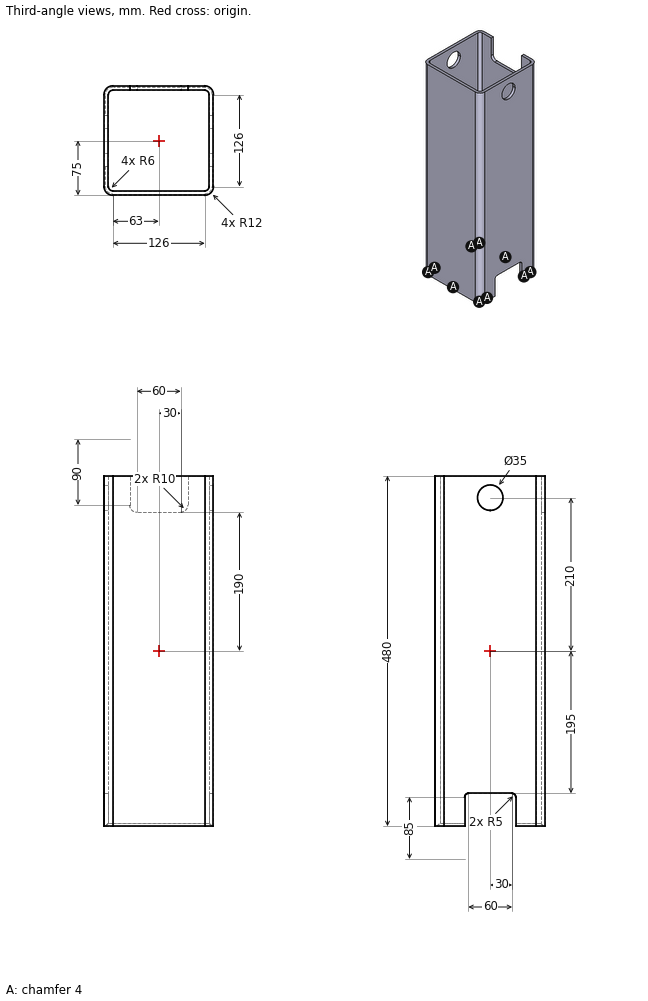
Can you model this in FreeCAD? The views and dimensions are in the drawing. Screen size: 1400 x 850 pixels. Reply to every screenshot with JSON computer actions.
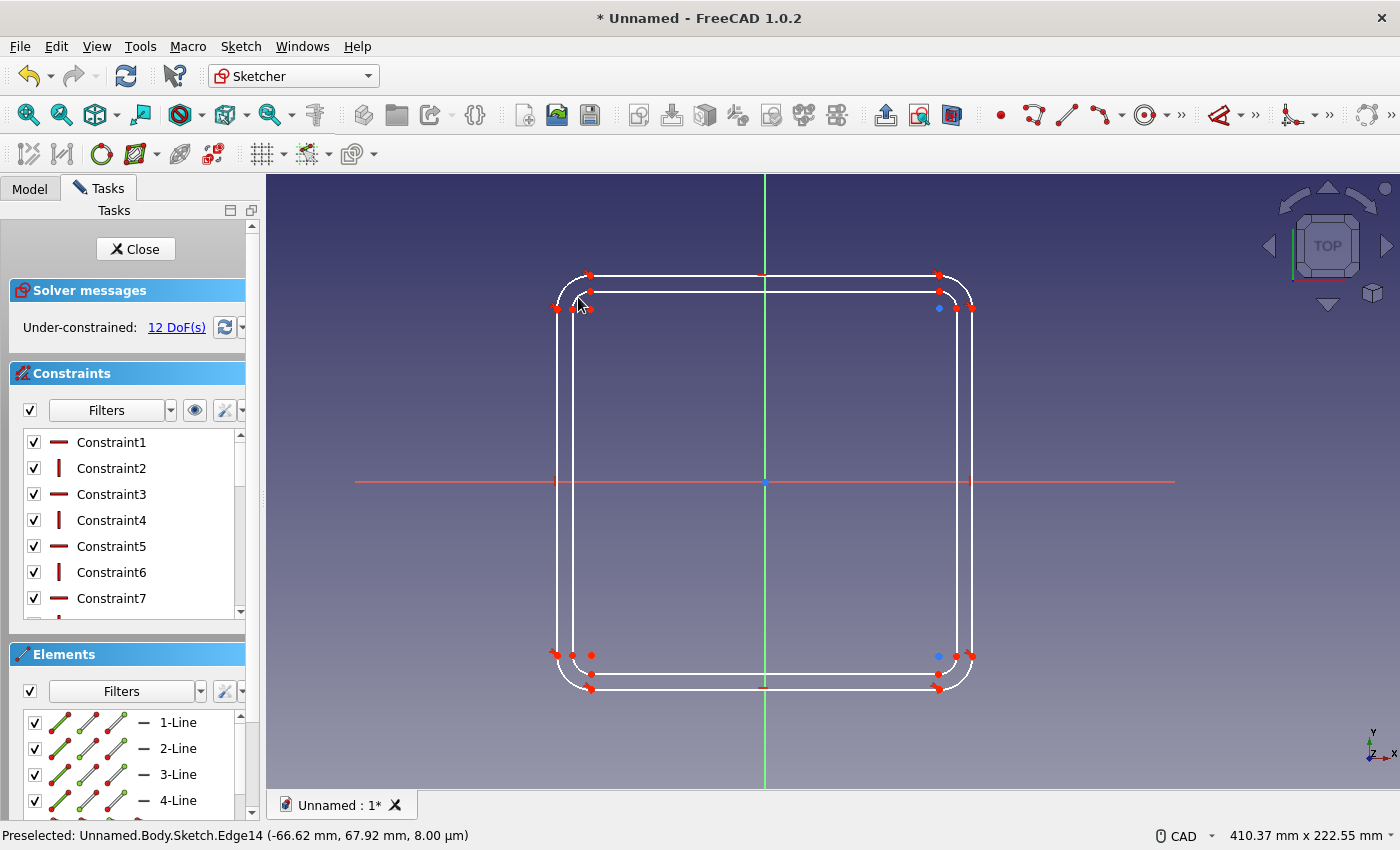
{"action": "left_click", "coordinate": [969, 294]}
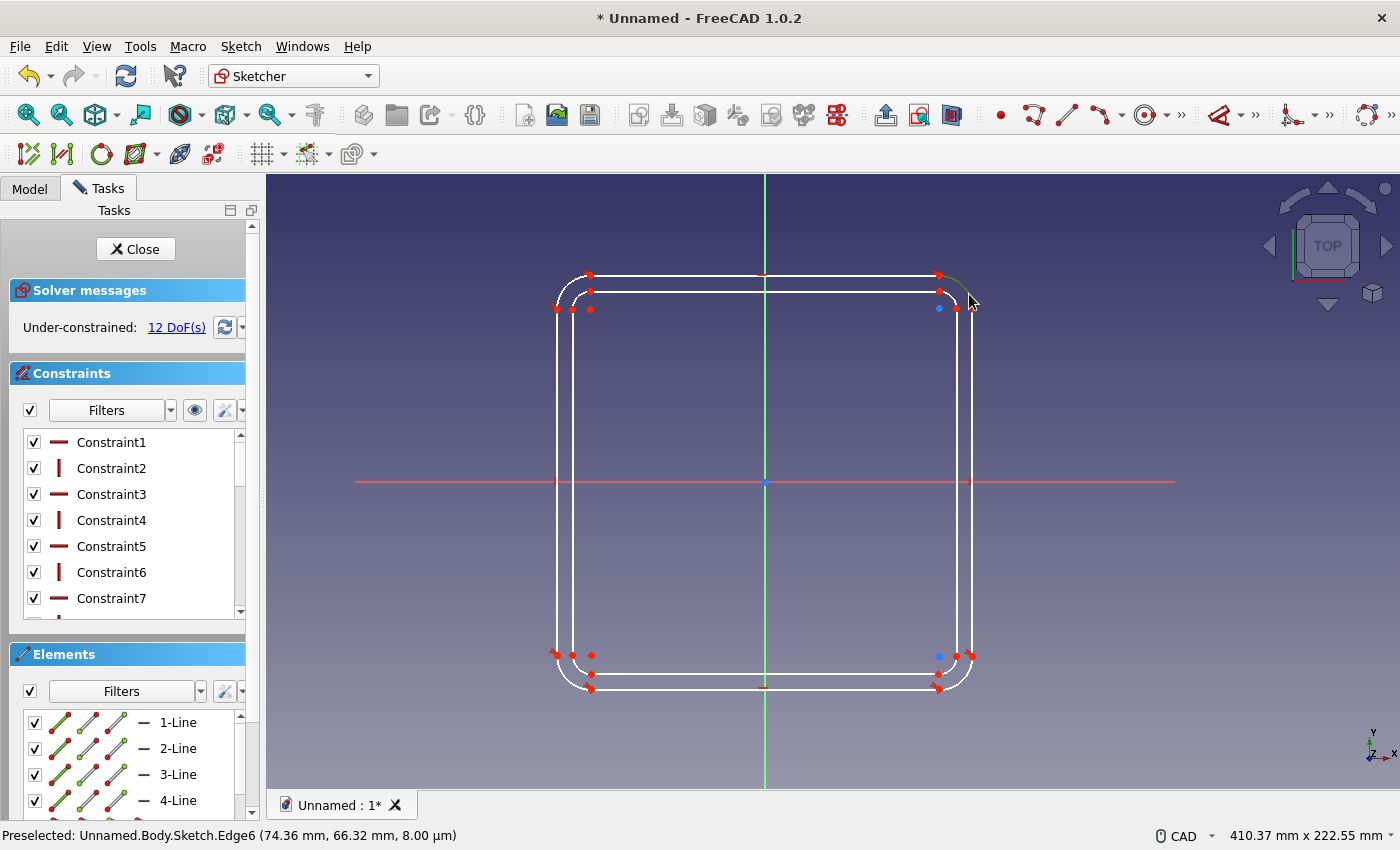
{"action": "left_click", "coordinate": [952, 297]}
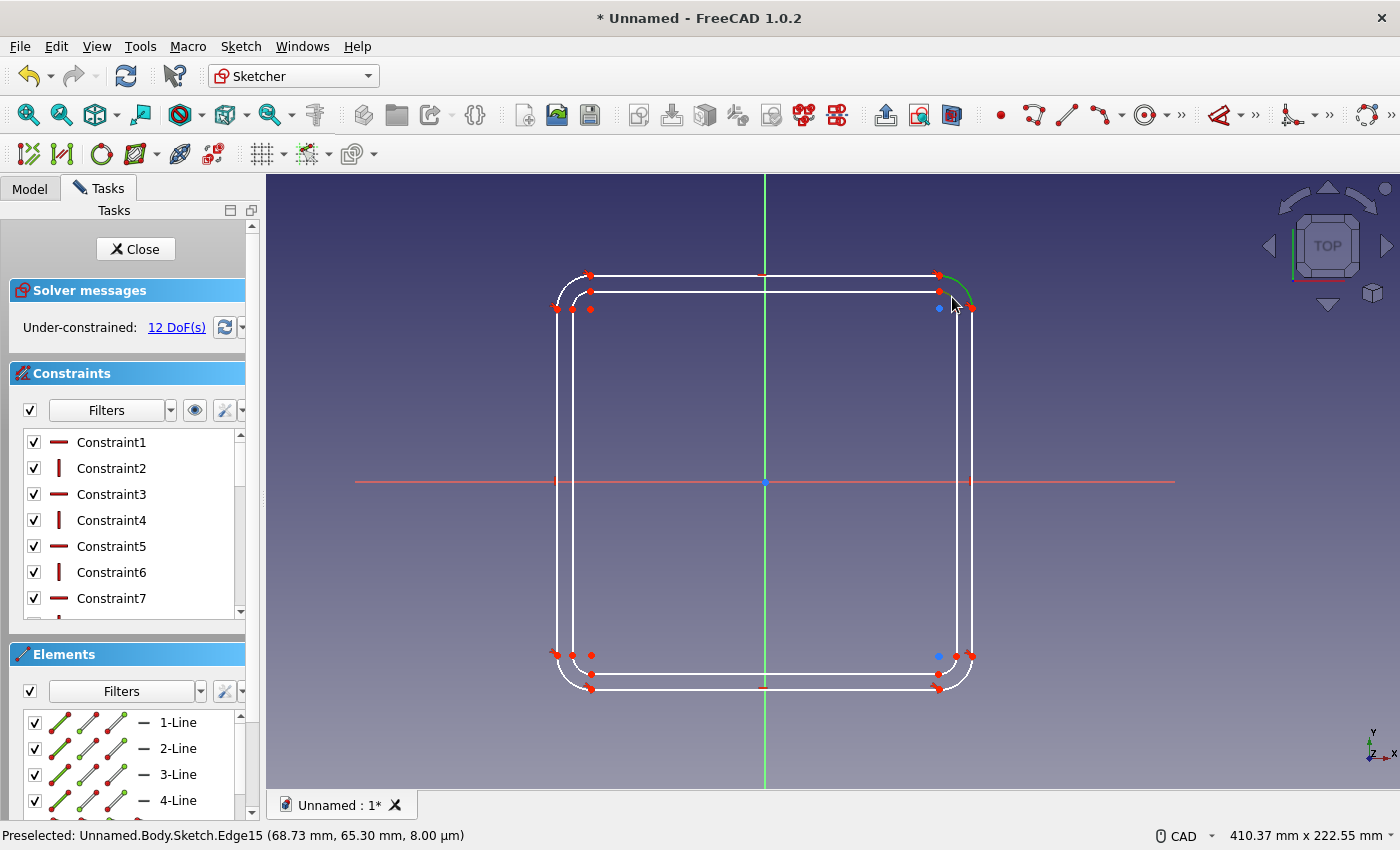
{"action": "key", "text": "c"}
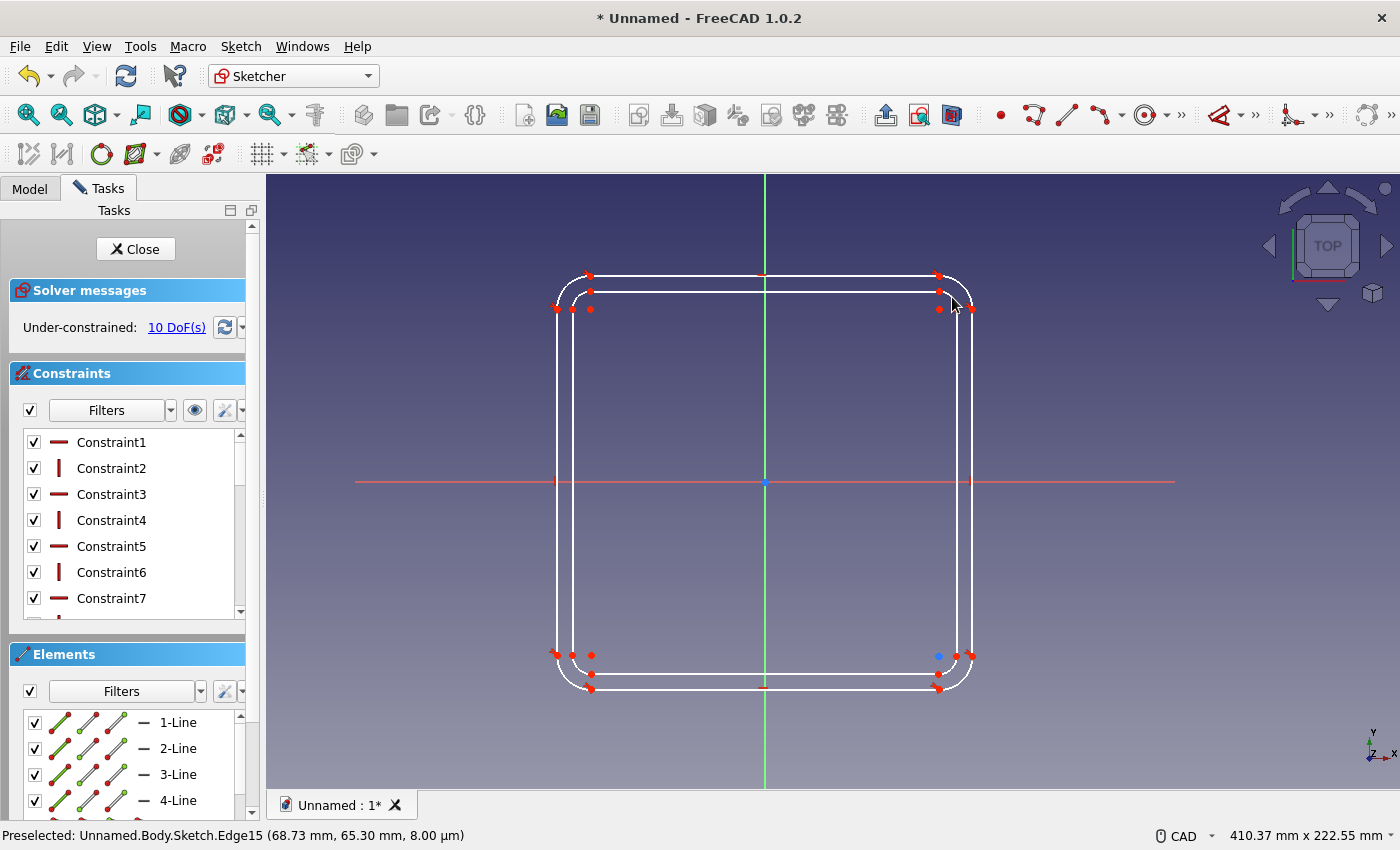
{"action": "left_click", "coordinate": [954, 686]}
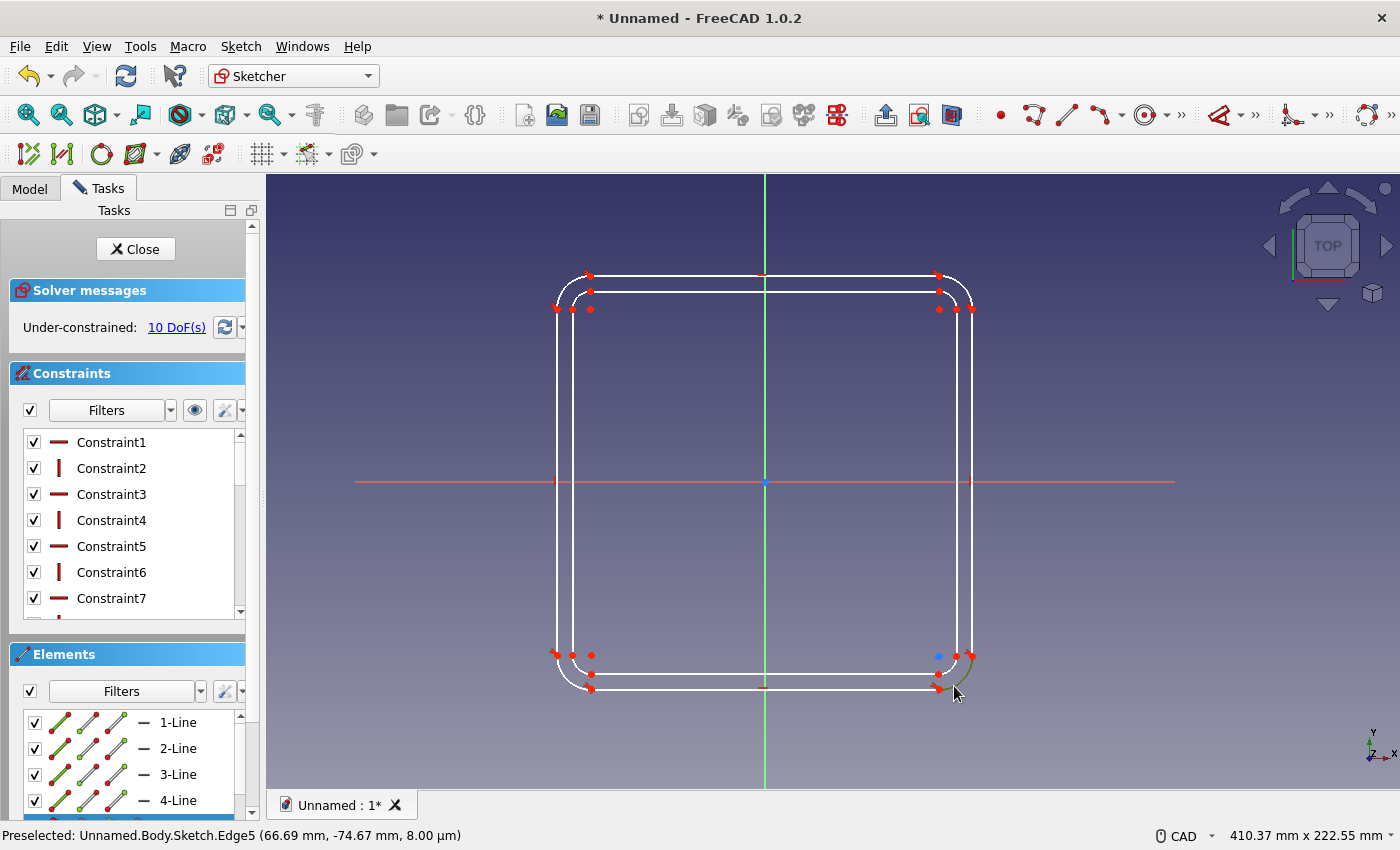
{"action": "left_click", "coordinate": [969, 294]}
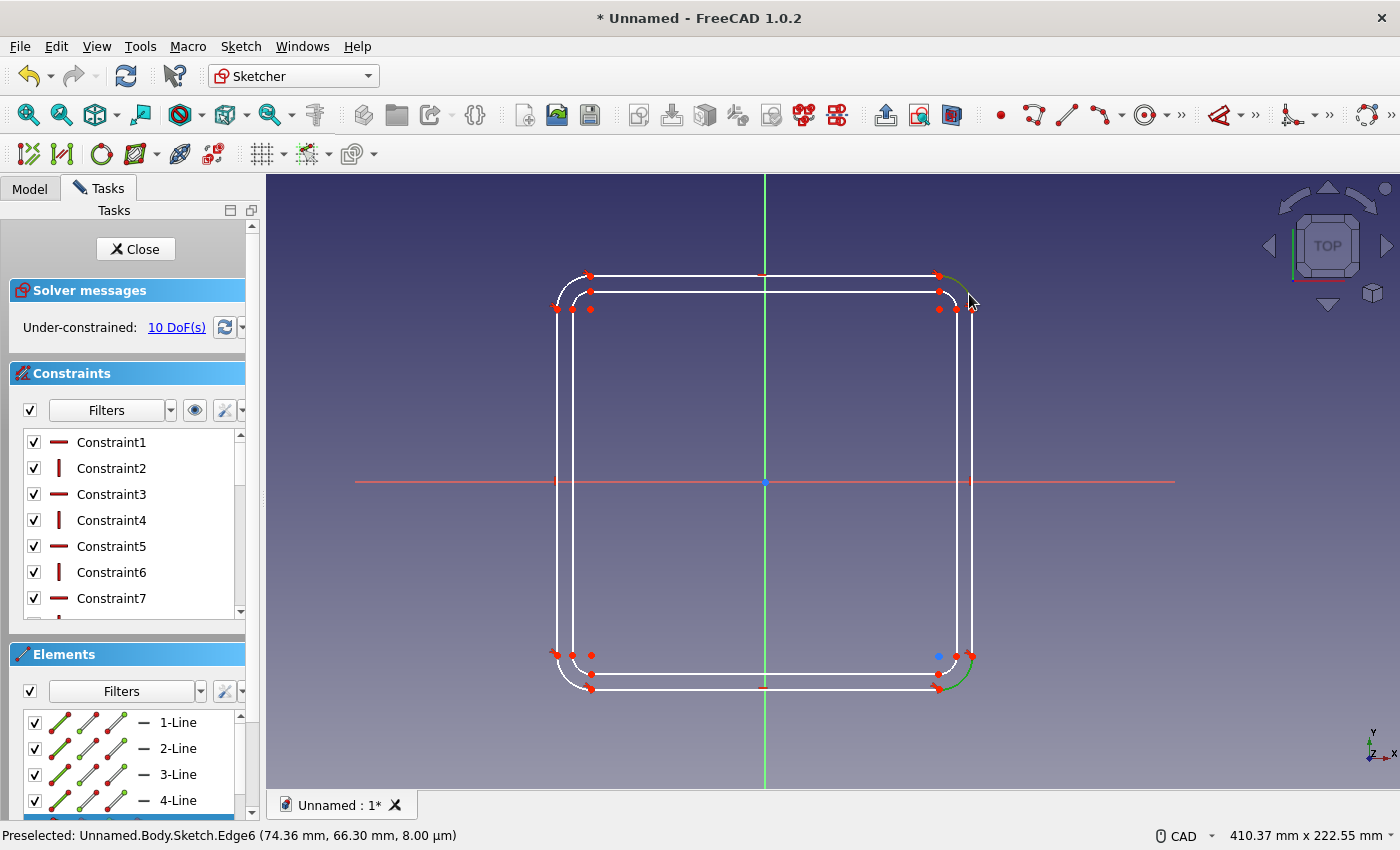
{"action": "left_click", "coordinate": [575, 280]}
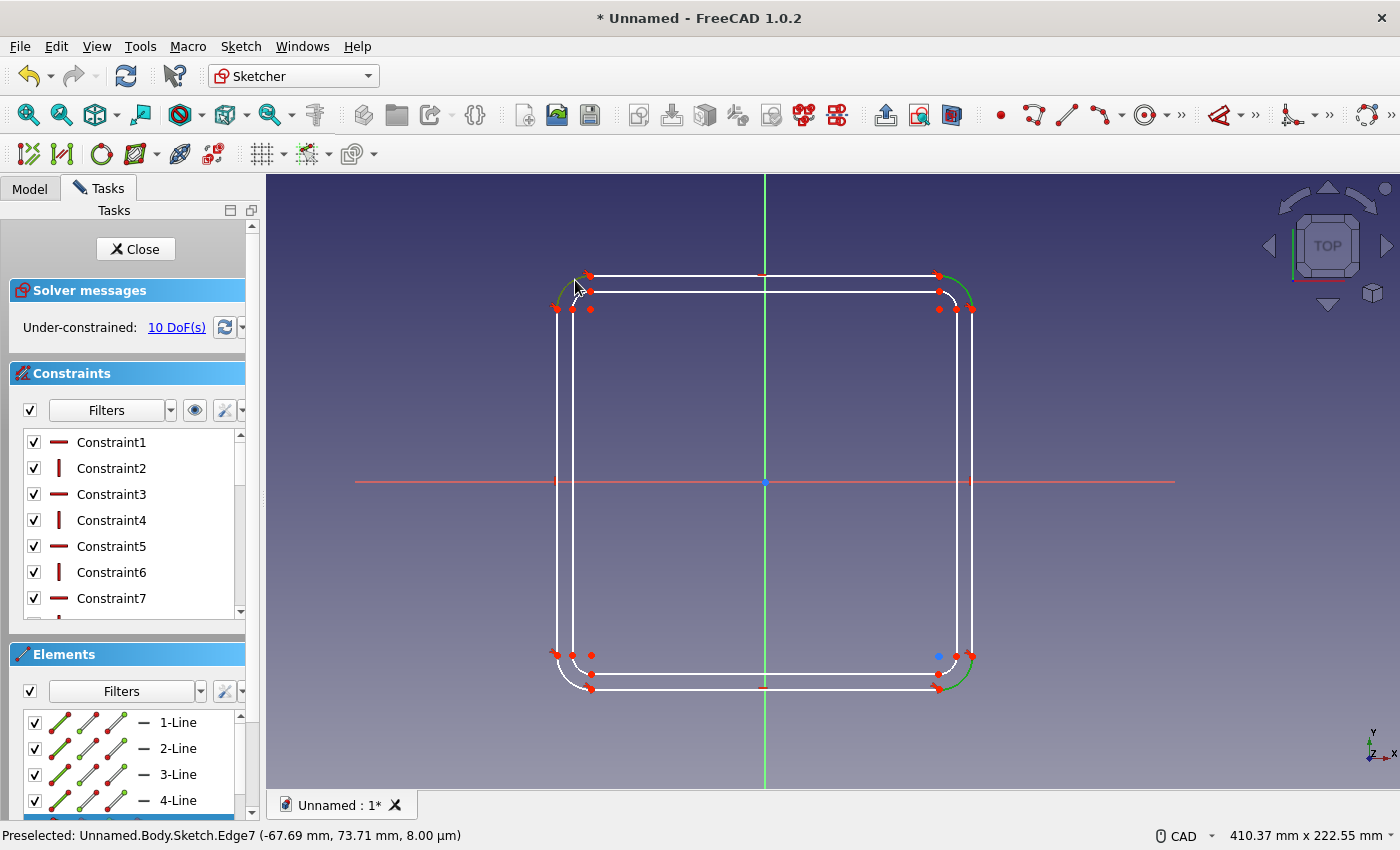
{"action": "left_click", "coordinate": [561, 671]}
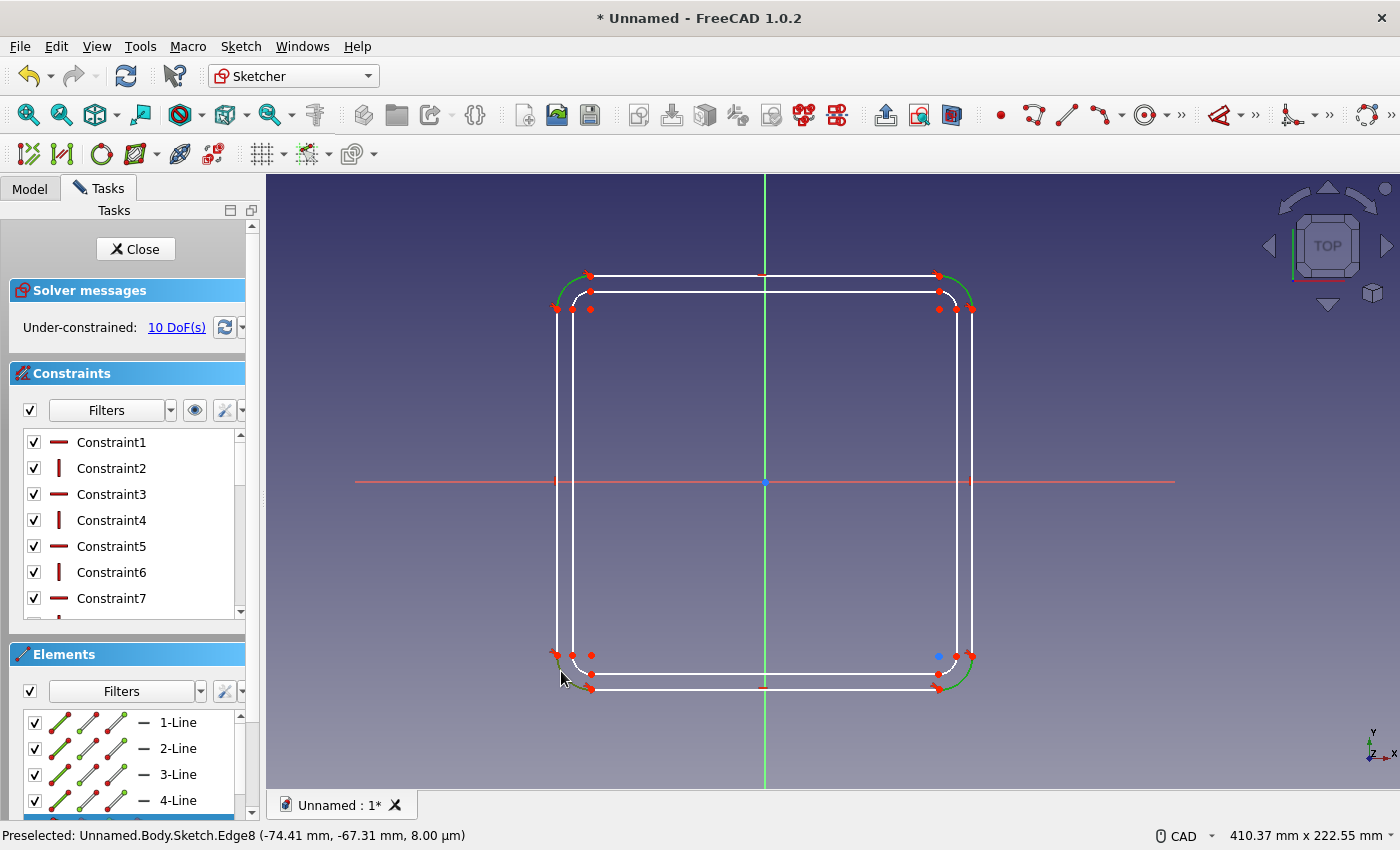
{"action": "key", "text": "e"}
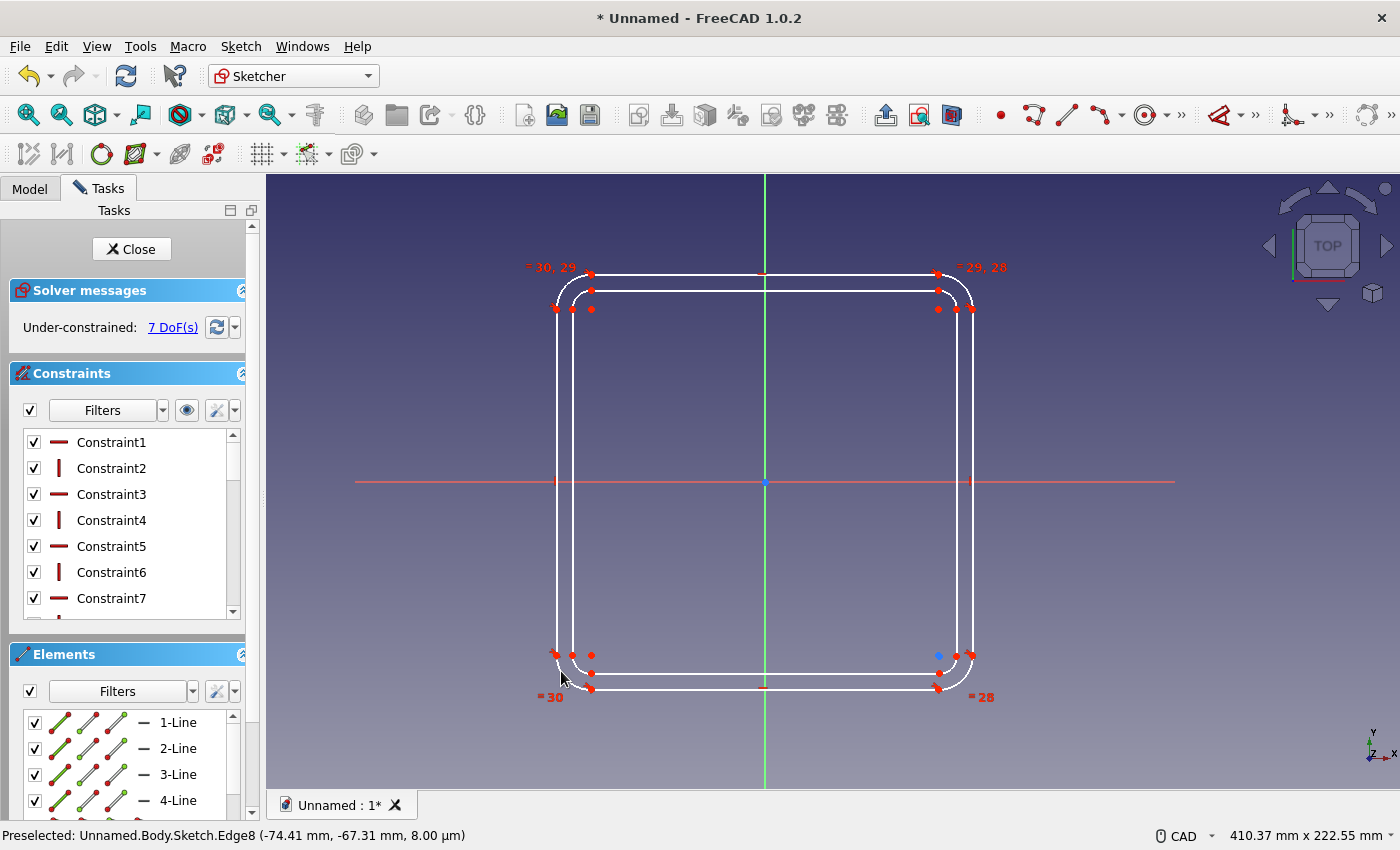
{"action": "left_click", "coordinate": [578, 669]}